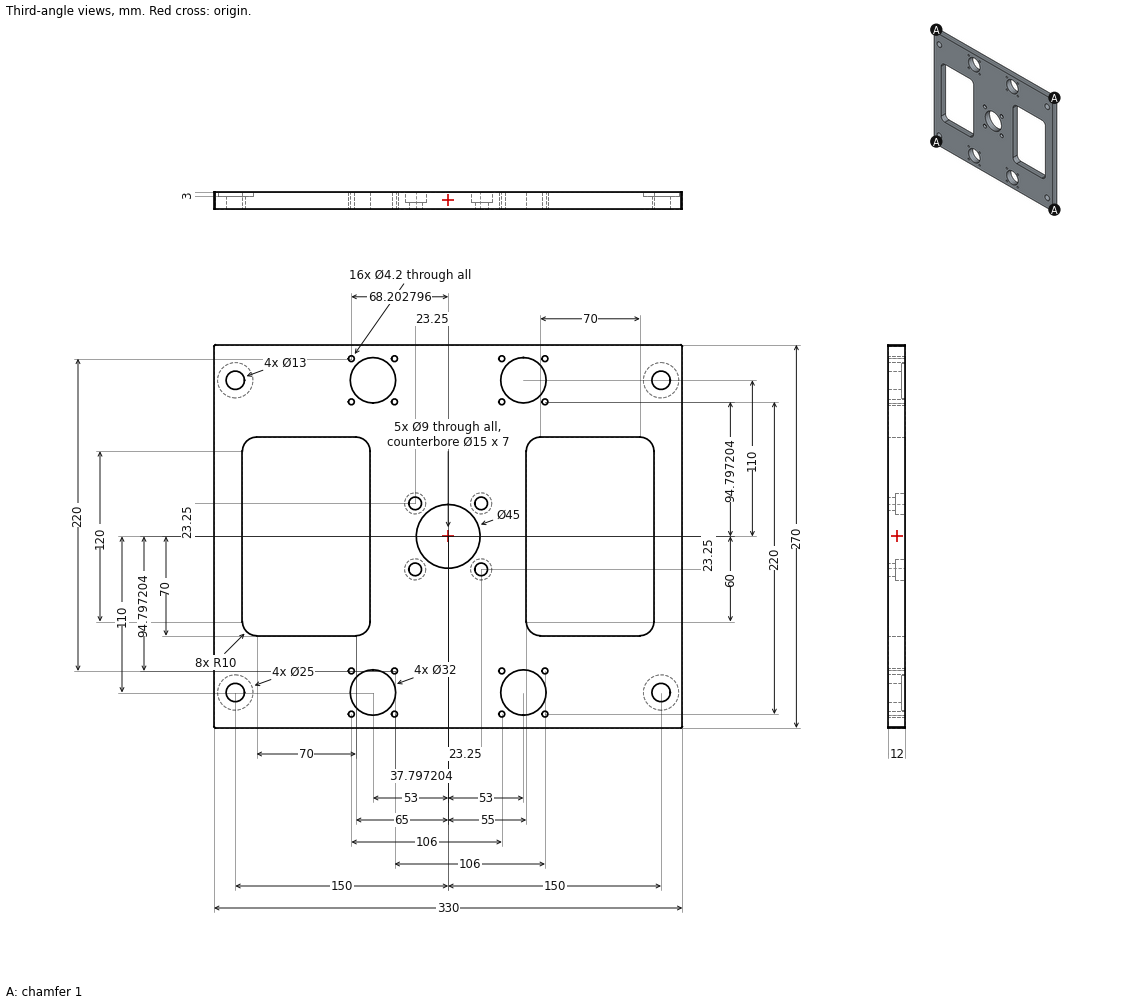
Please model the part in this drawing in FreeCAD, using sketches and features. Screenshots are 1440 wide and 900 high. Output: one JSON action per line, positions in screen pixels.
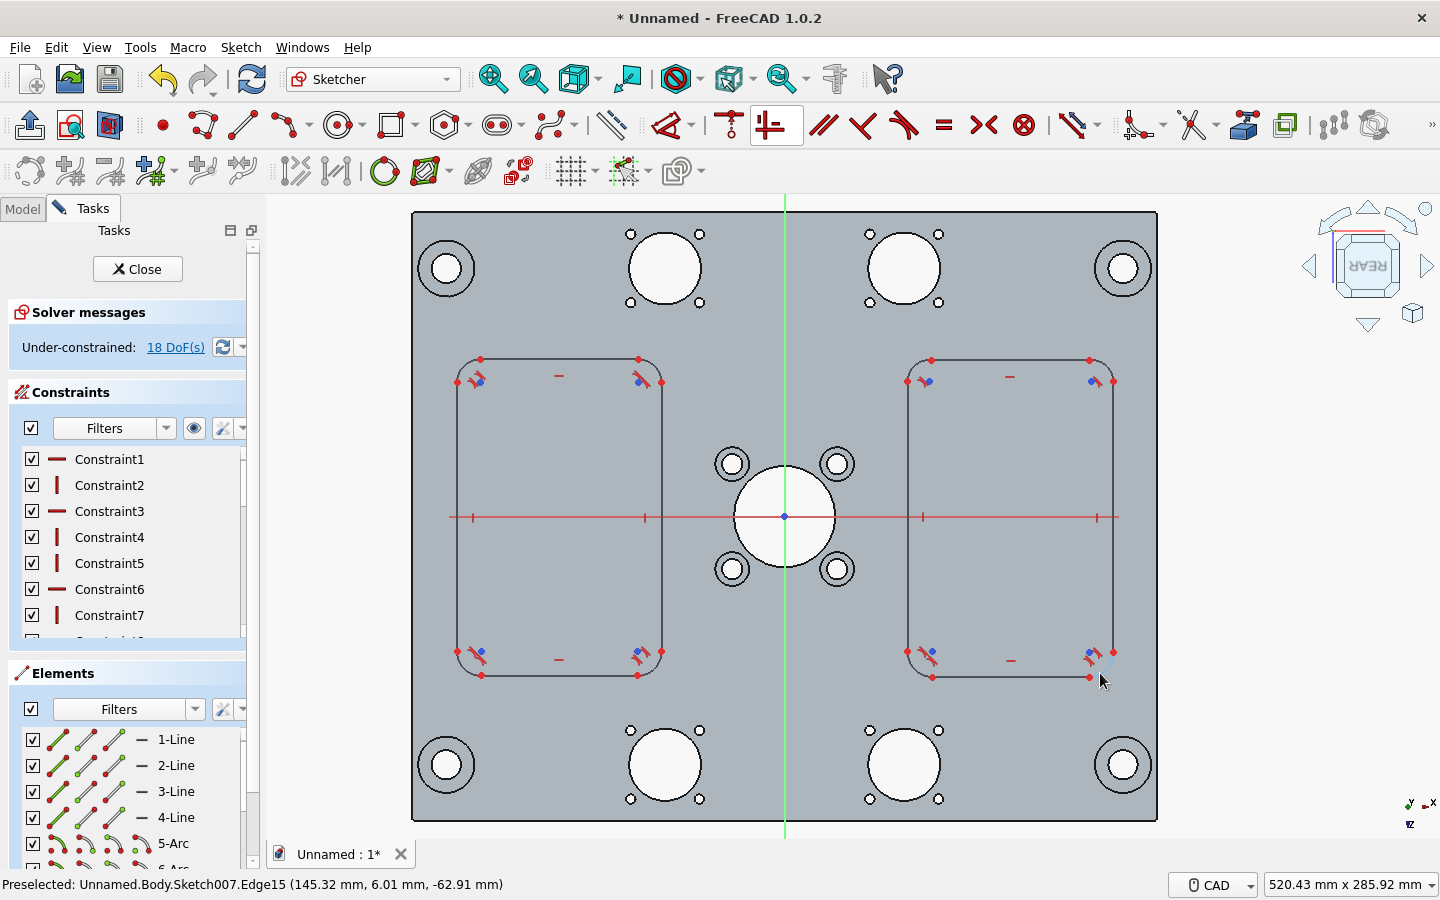
{"action": "left_click", "coordinate": [1042, 360]}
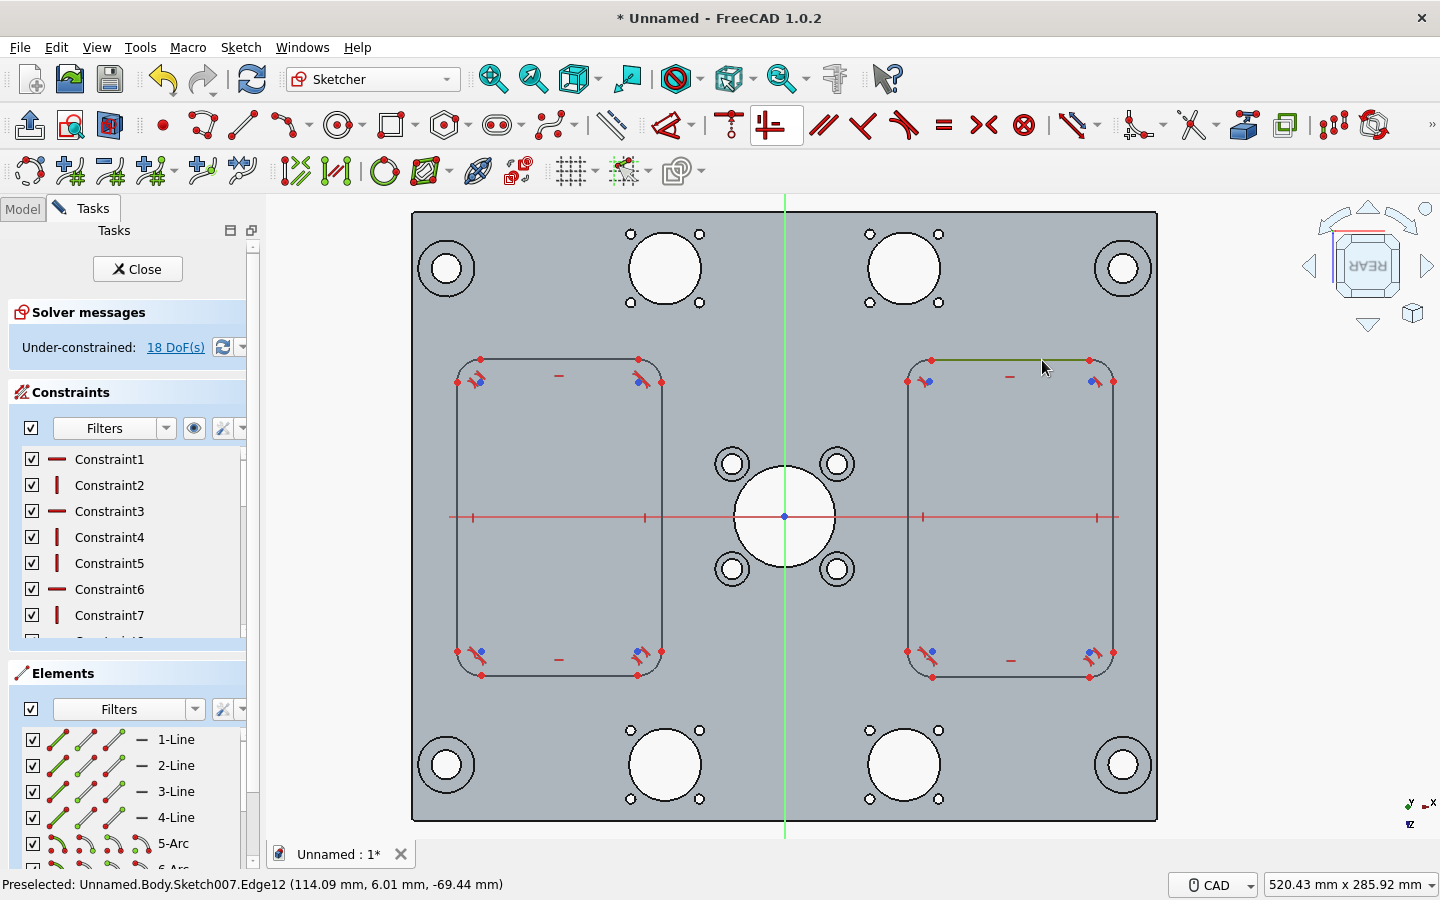
{"action": "scroll", "coordinate": [1111, 372], "scroll_direction": "up", "scroll_amount": 2}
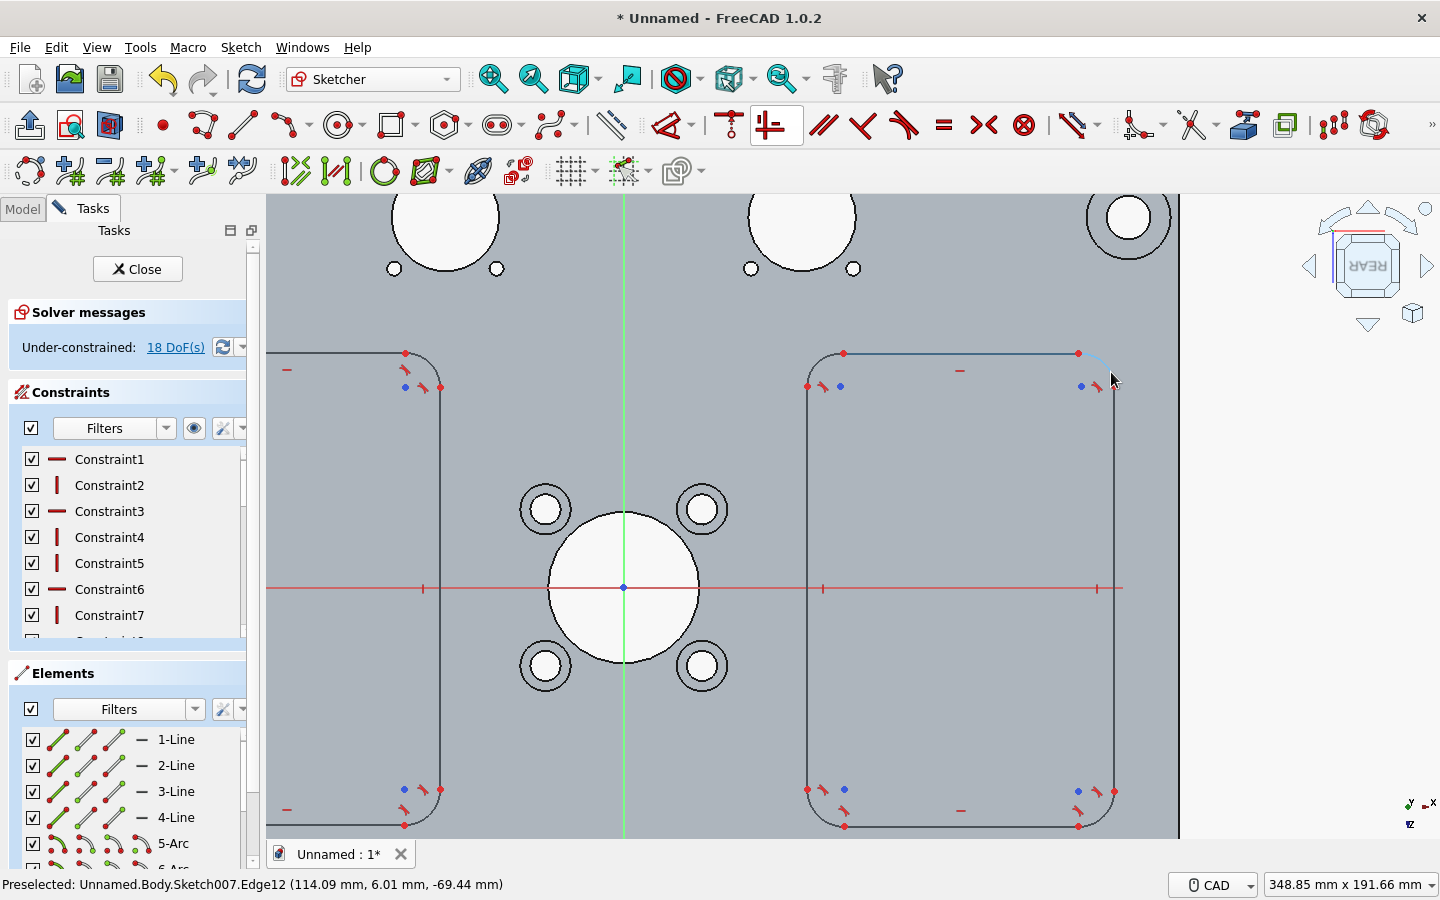
{"action": "left_click", "coordinate": [1110, 371]}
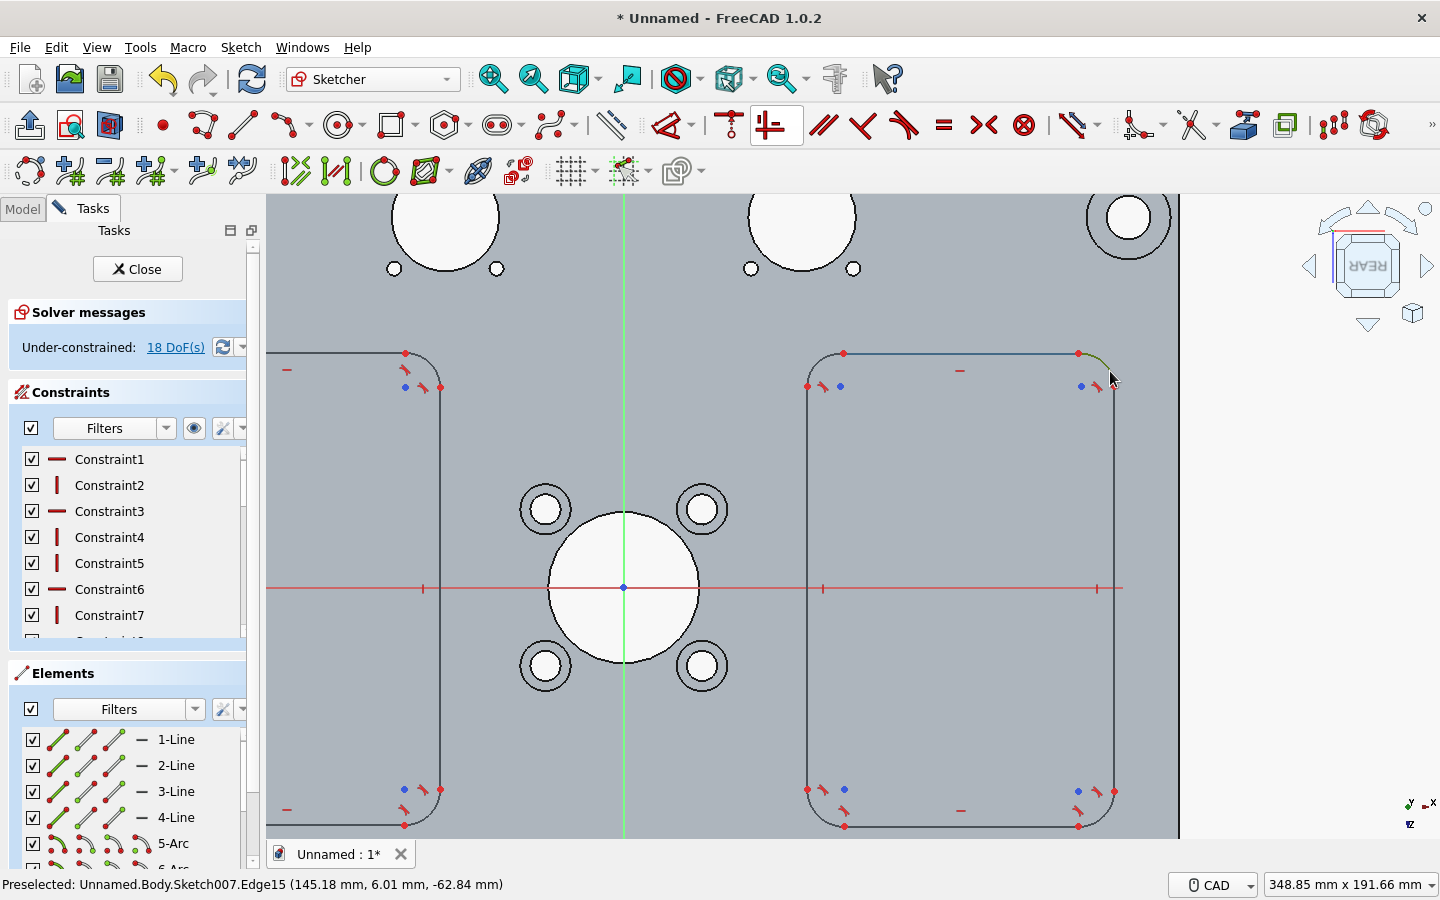
{"action": "key", "text": "t"}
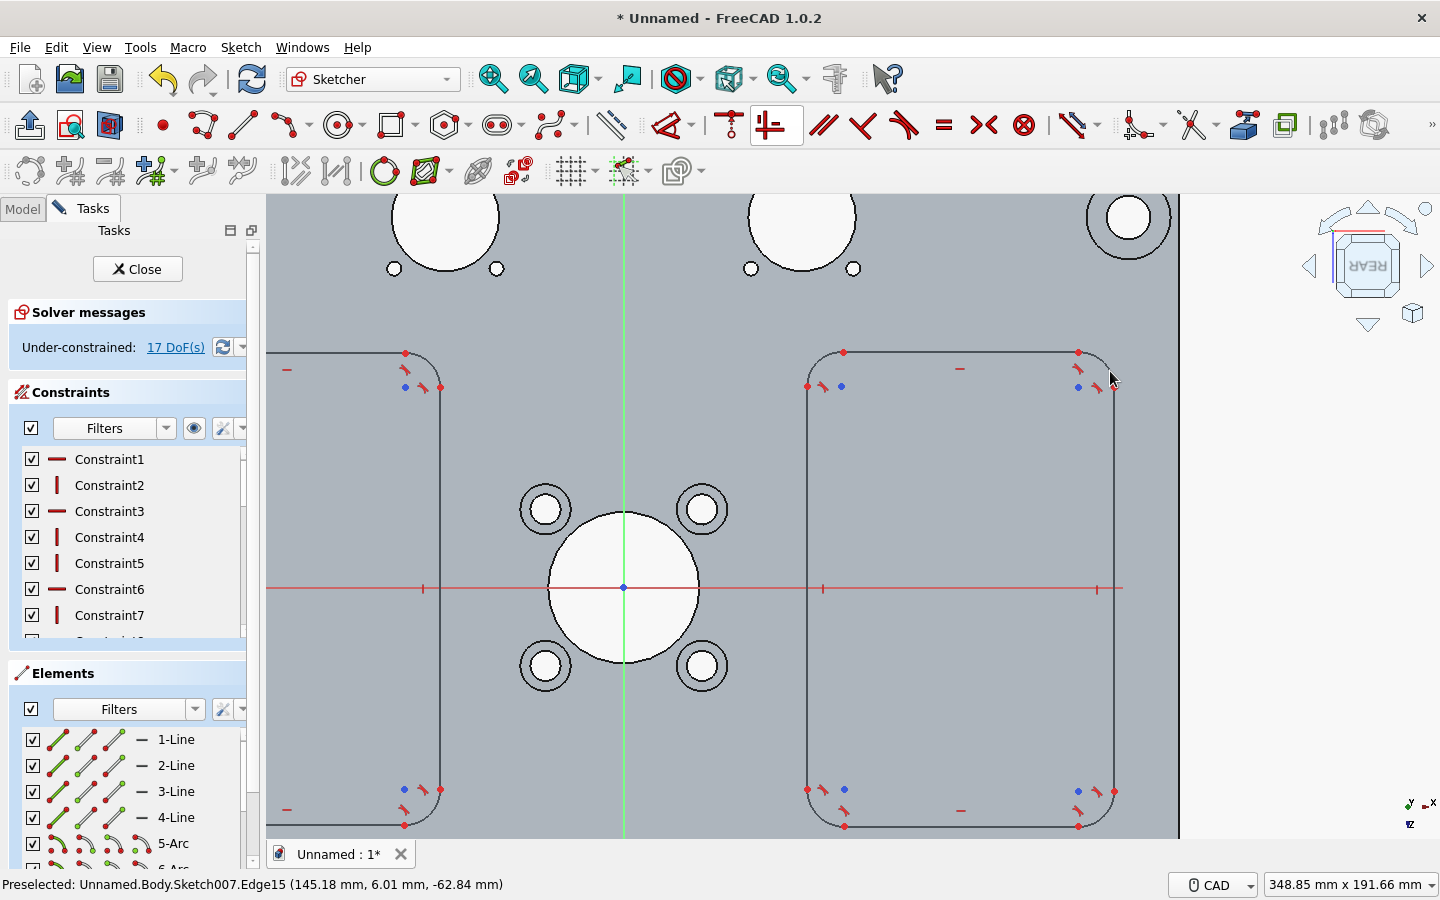
{"action": "left_click", "coordinate": [1008, 352]}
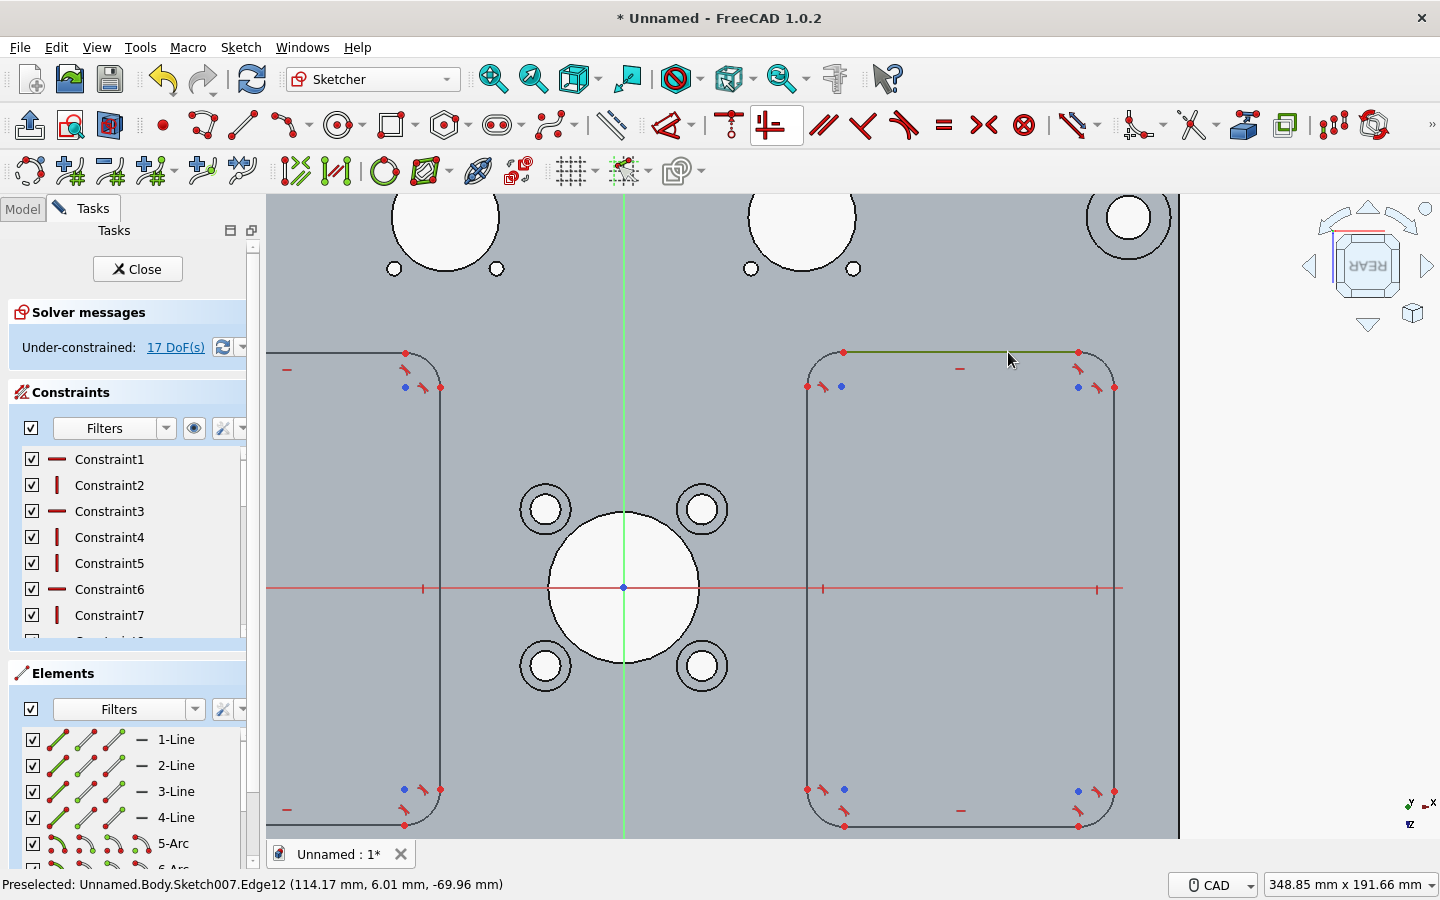
{"action": "left_click", "coordinate": [827, 356]}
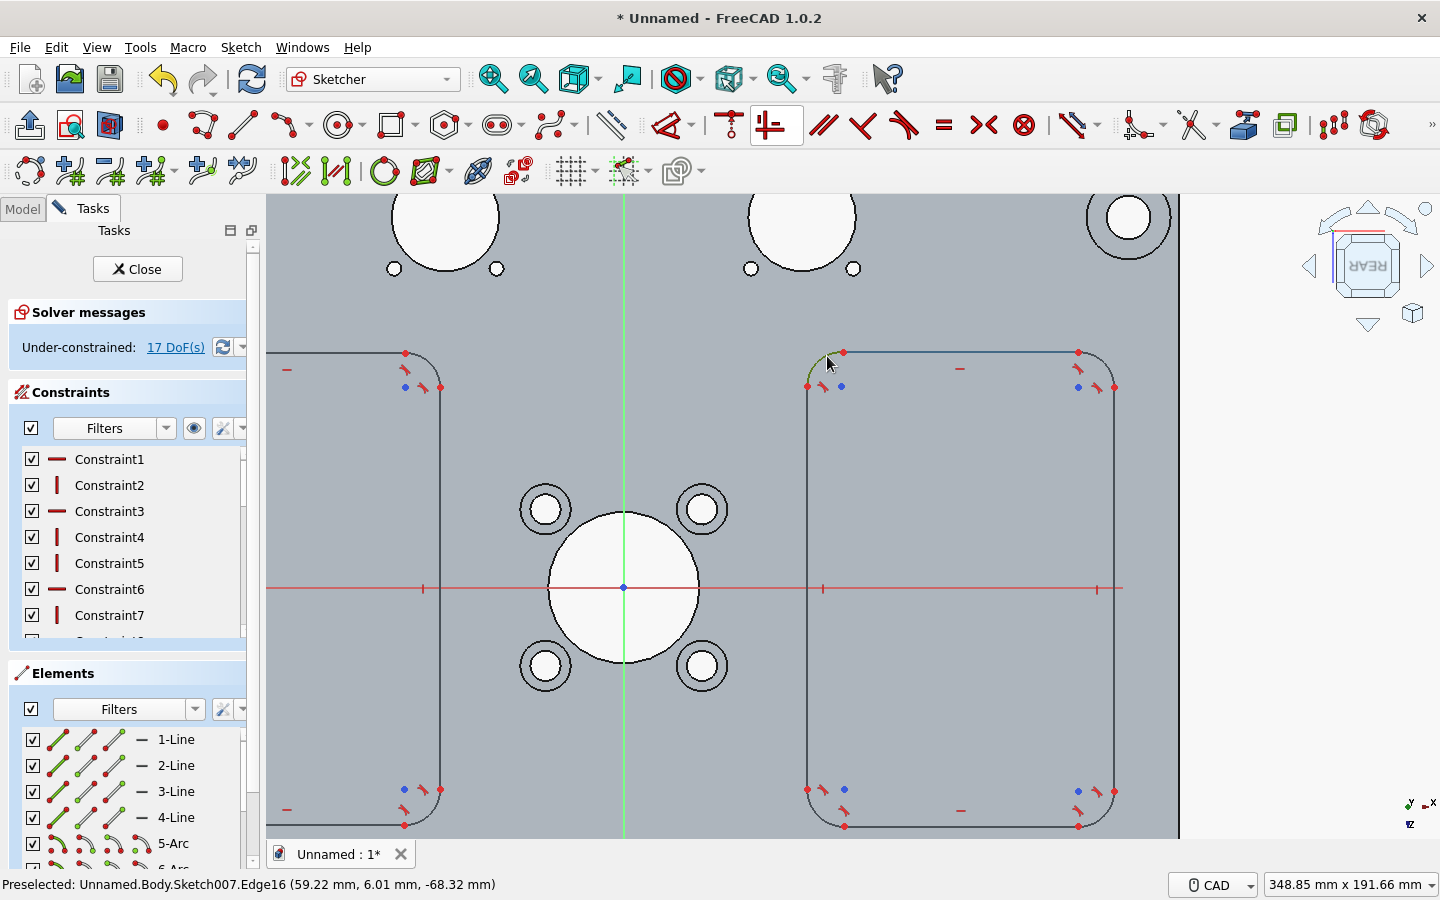
{"action": "left_click", "coordinate": [904, 126]}